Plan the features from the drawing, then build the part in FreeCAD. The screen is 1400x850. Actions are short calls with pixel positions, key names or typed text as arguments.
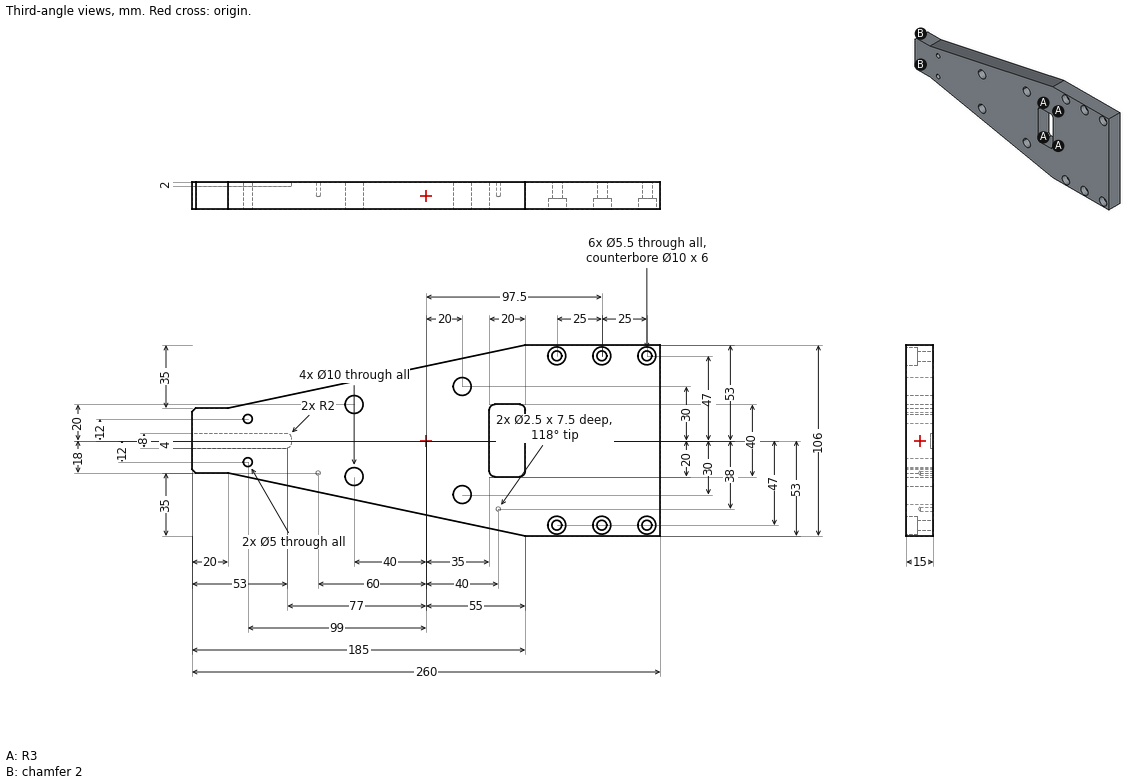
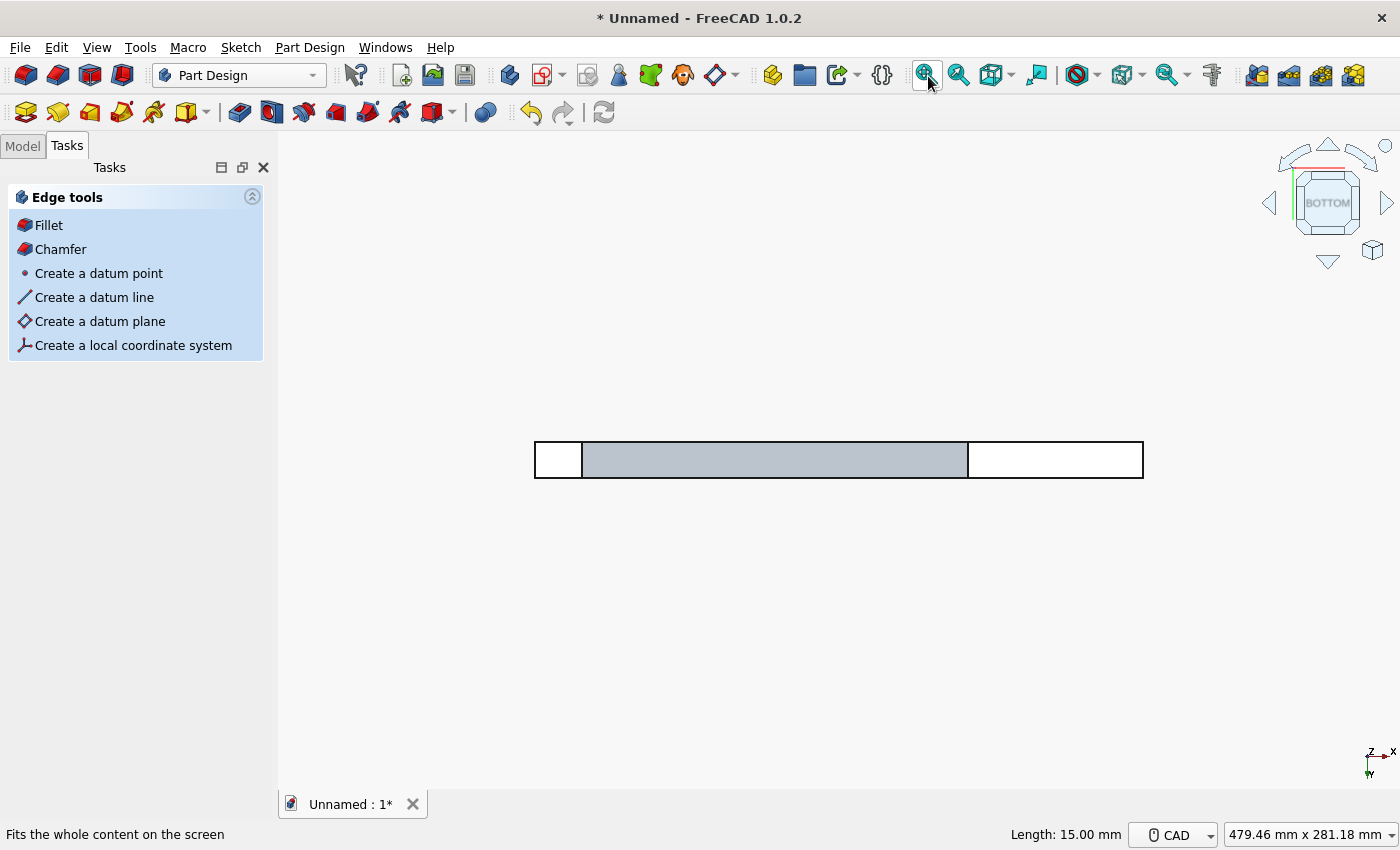
click(535, 459, ctrl)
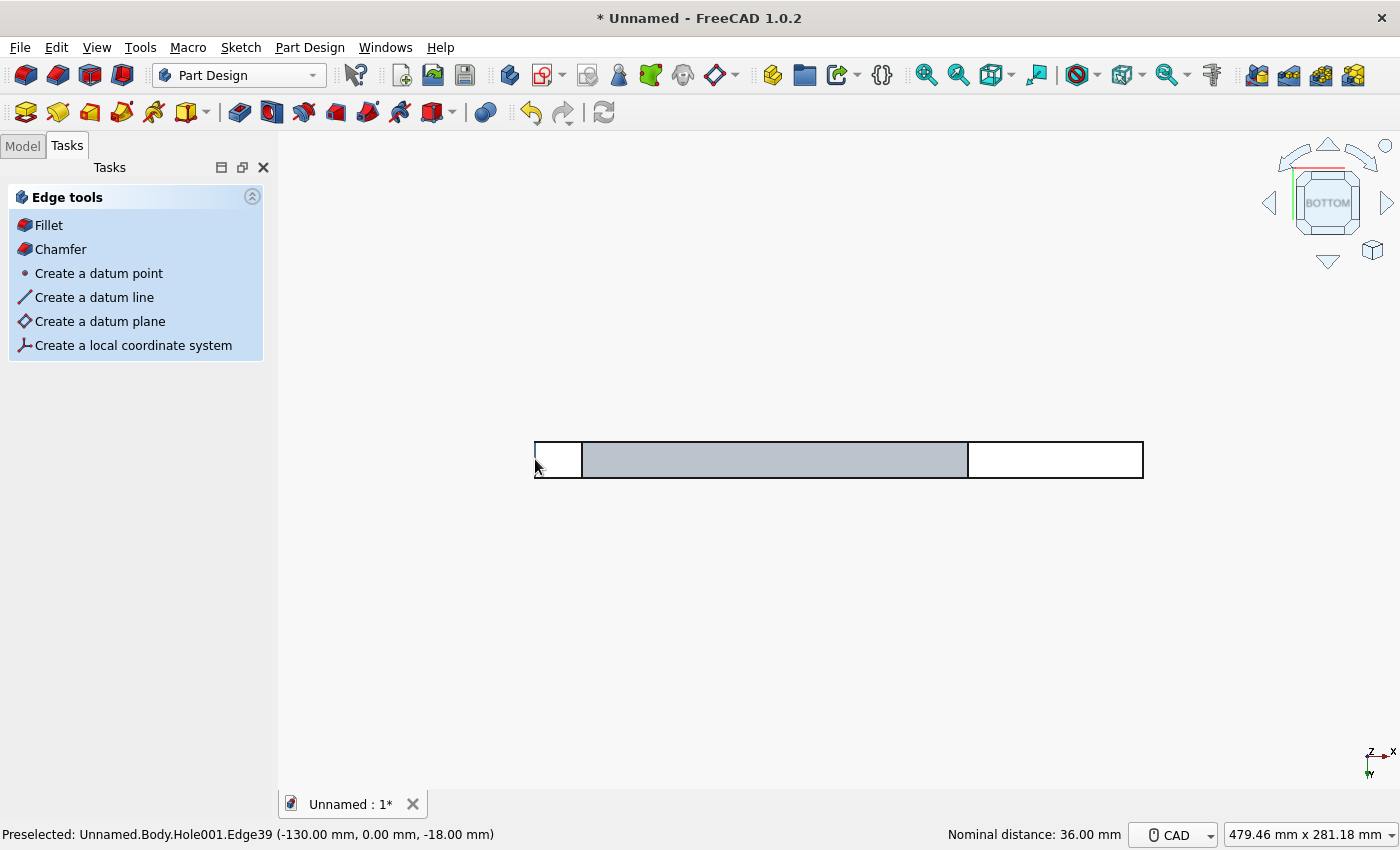
click(58, 76)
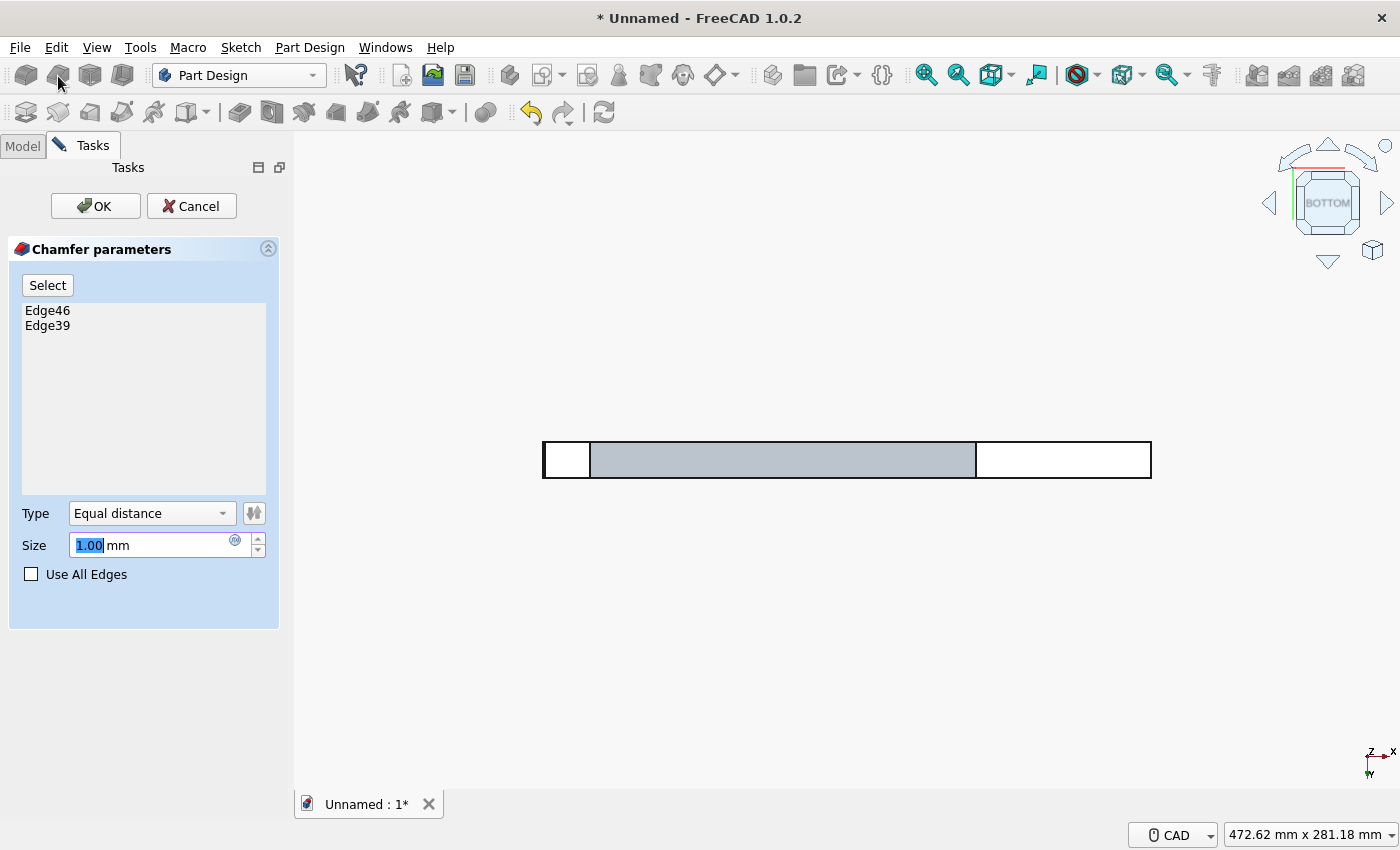
text(2)
key(Tab)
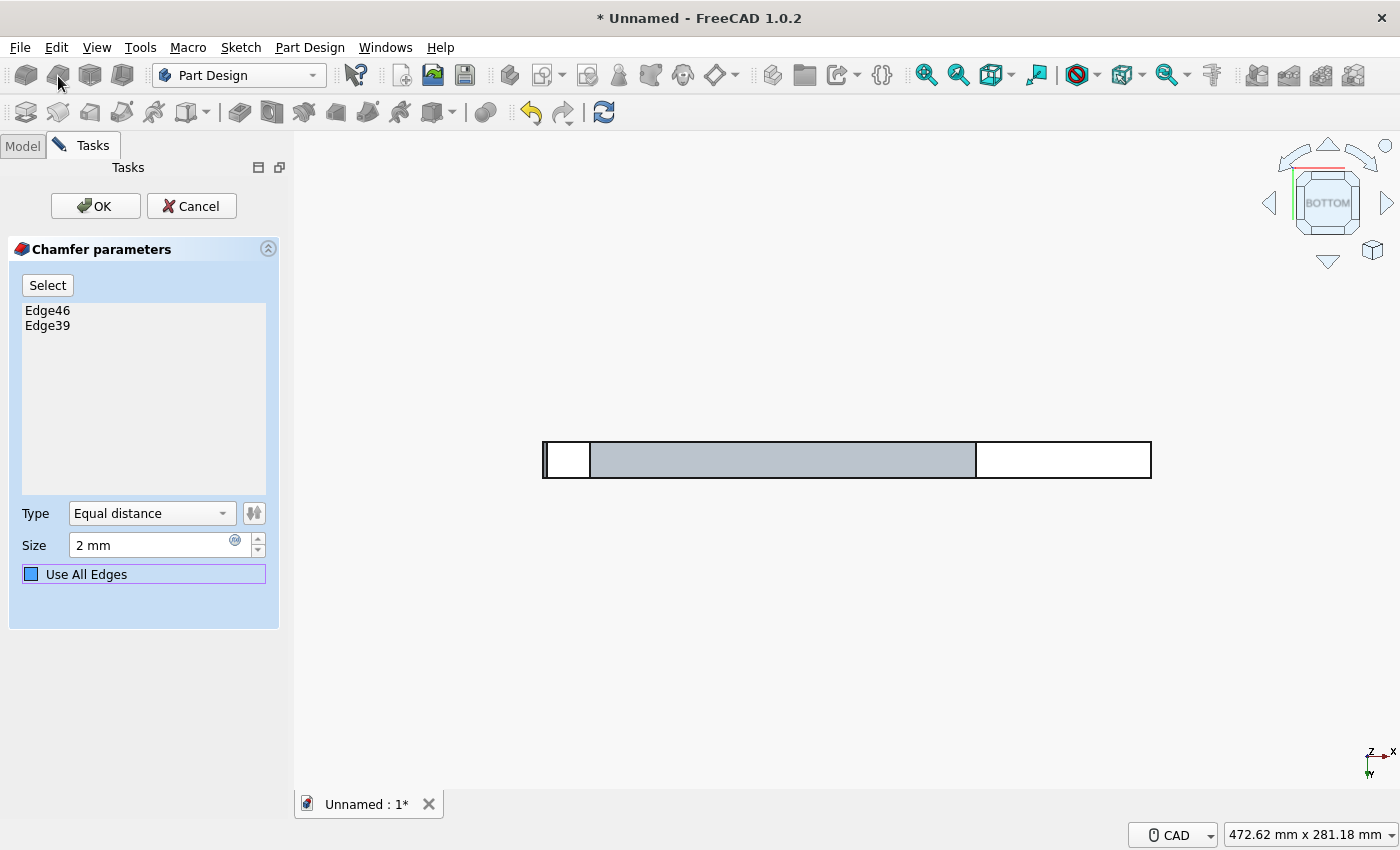
click(96, 206)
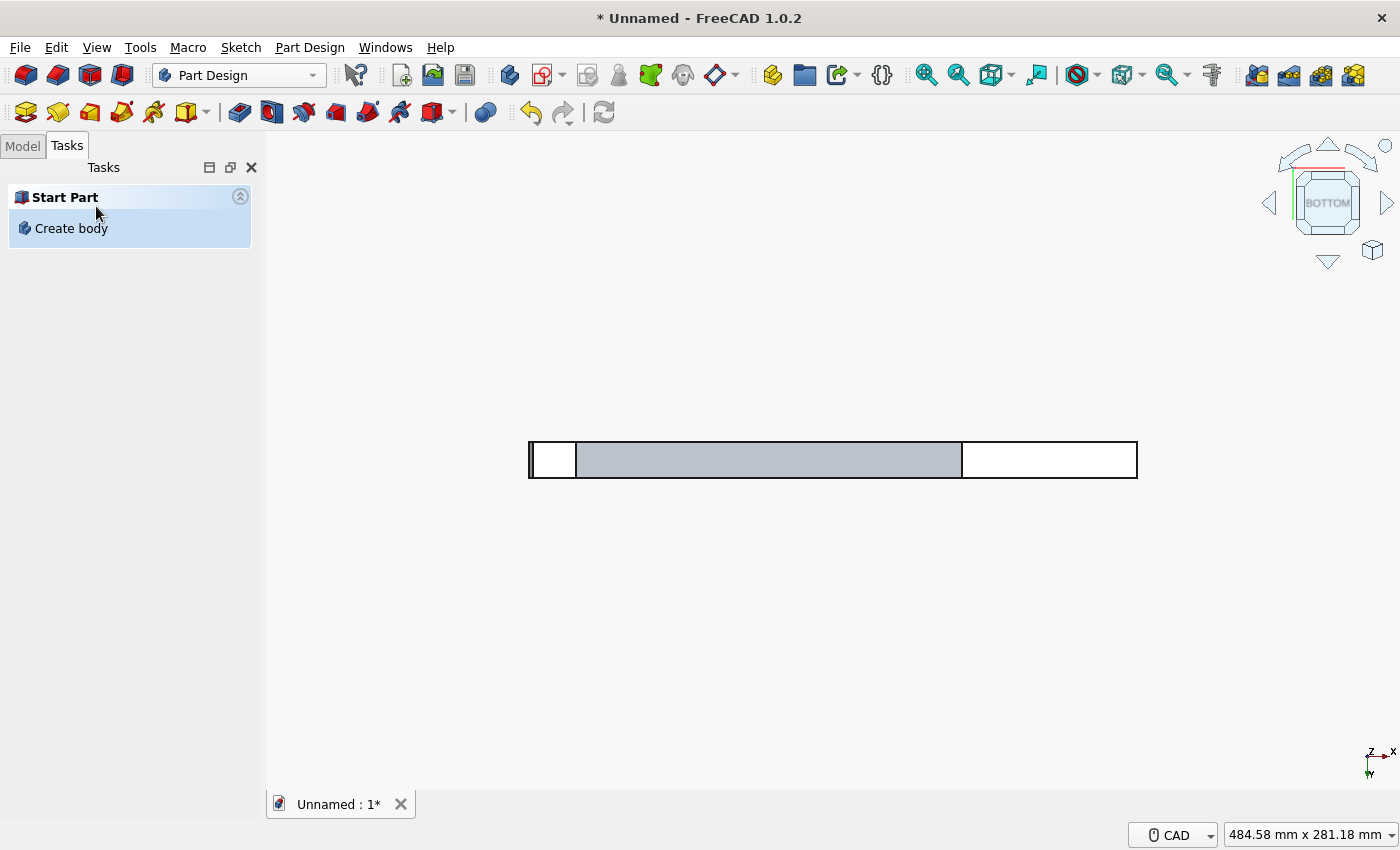
key(4)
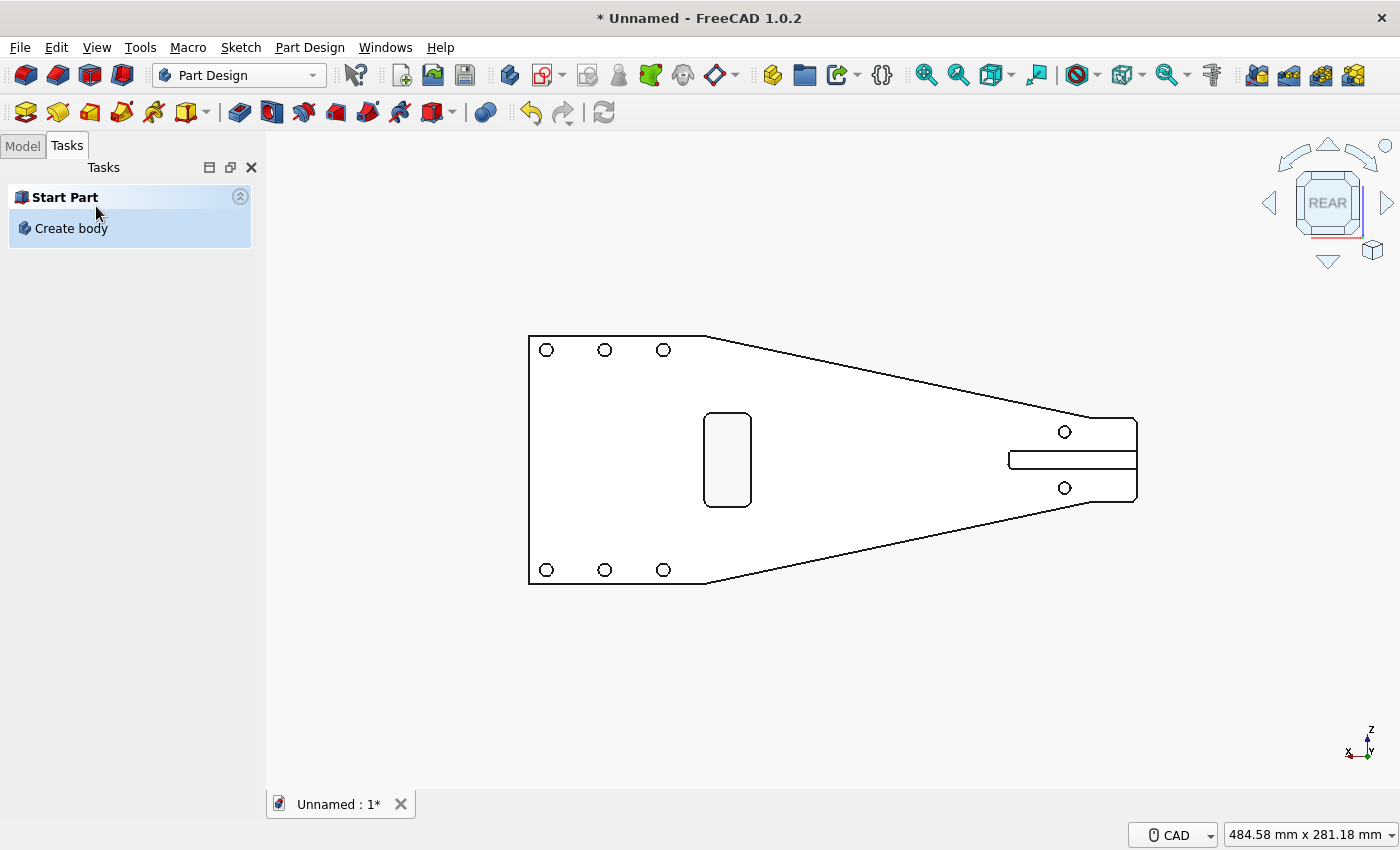
click(833, 459)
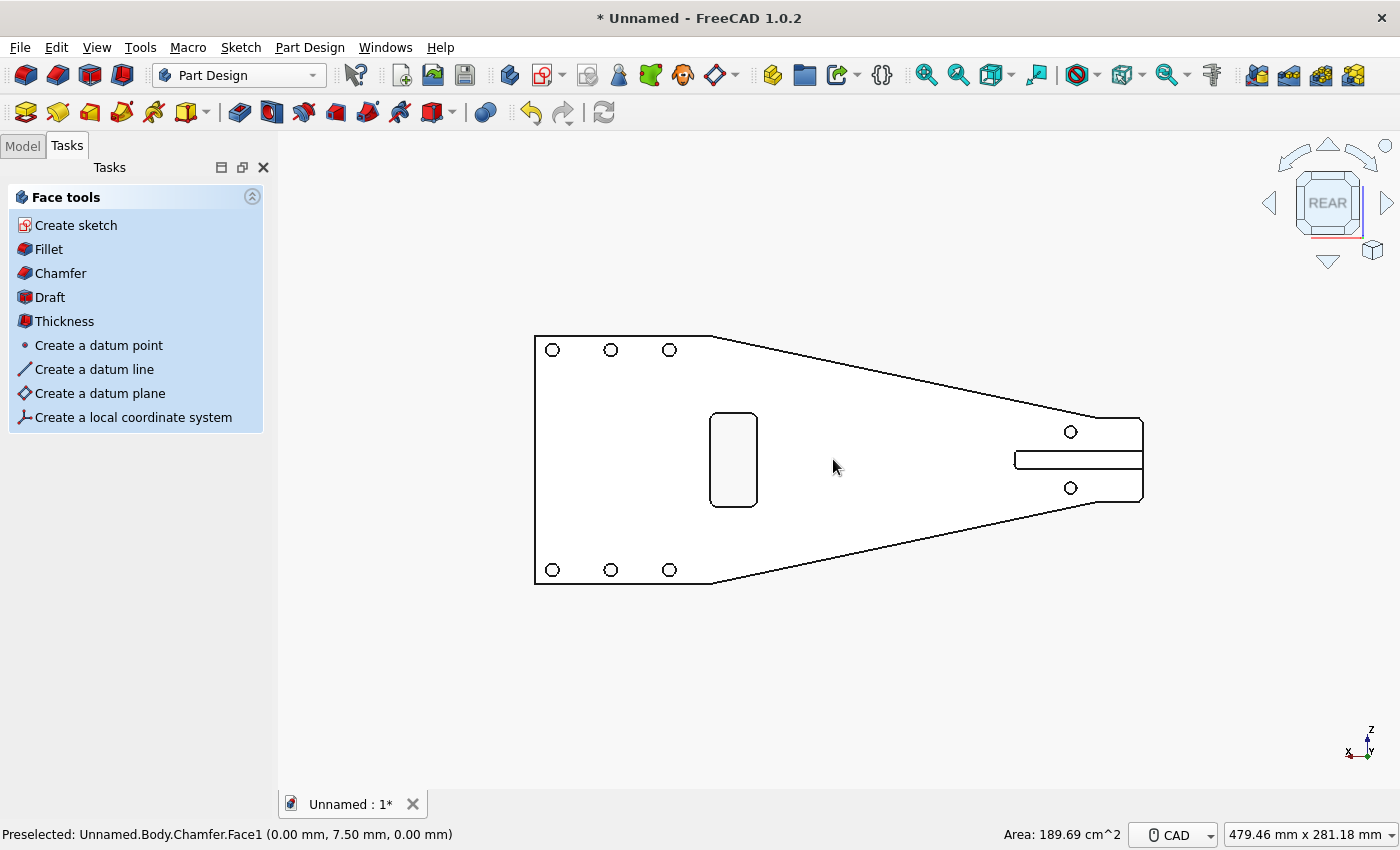
click(542, 76)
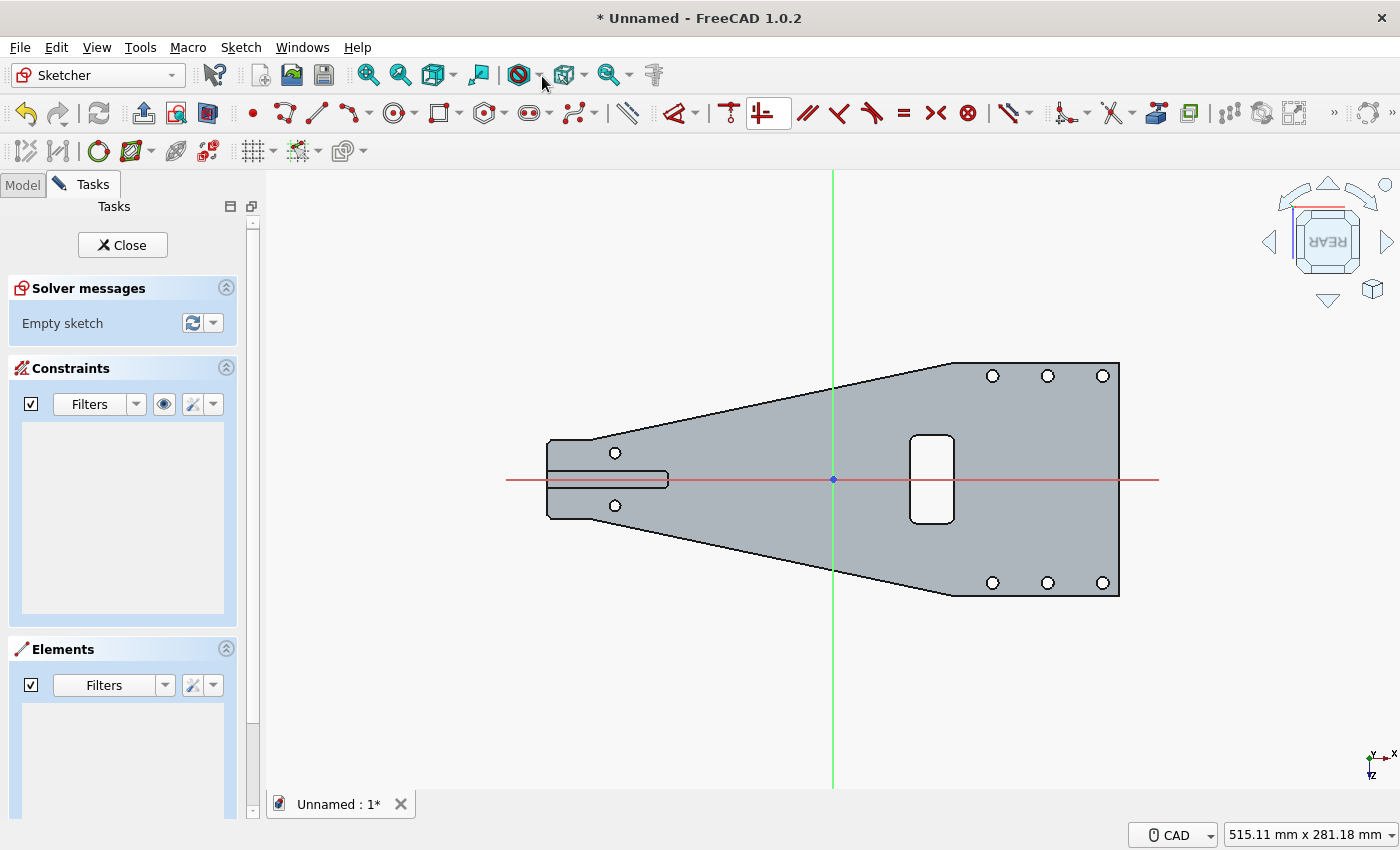
scroll(838, 411, up, 5)